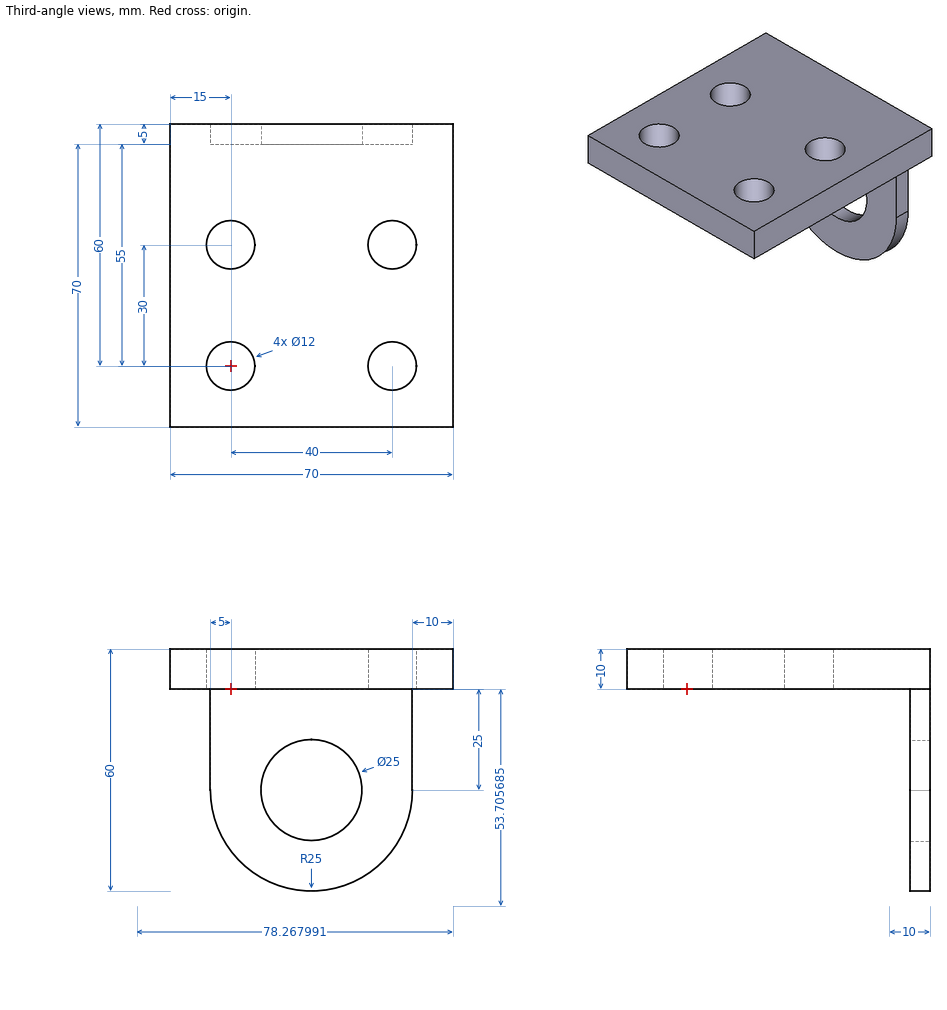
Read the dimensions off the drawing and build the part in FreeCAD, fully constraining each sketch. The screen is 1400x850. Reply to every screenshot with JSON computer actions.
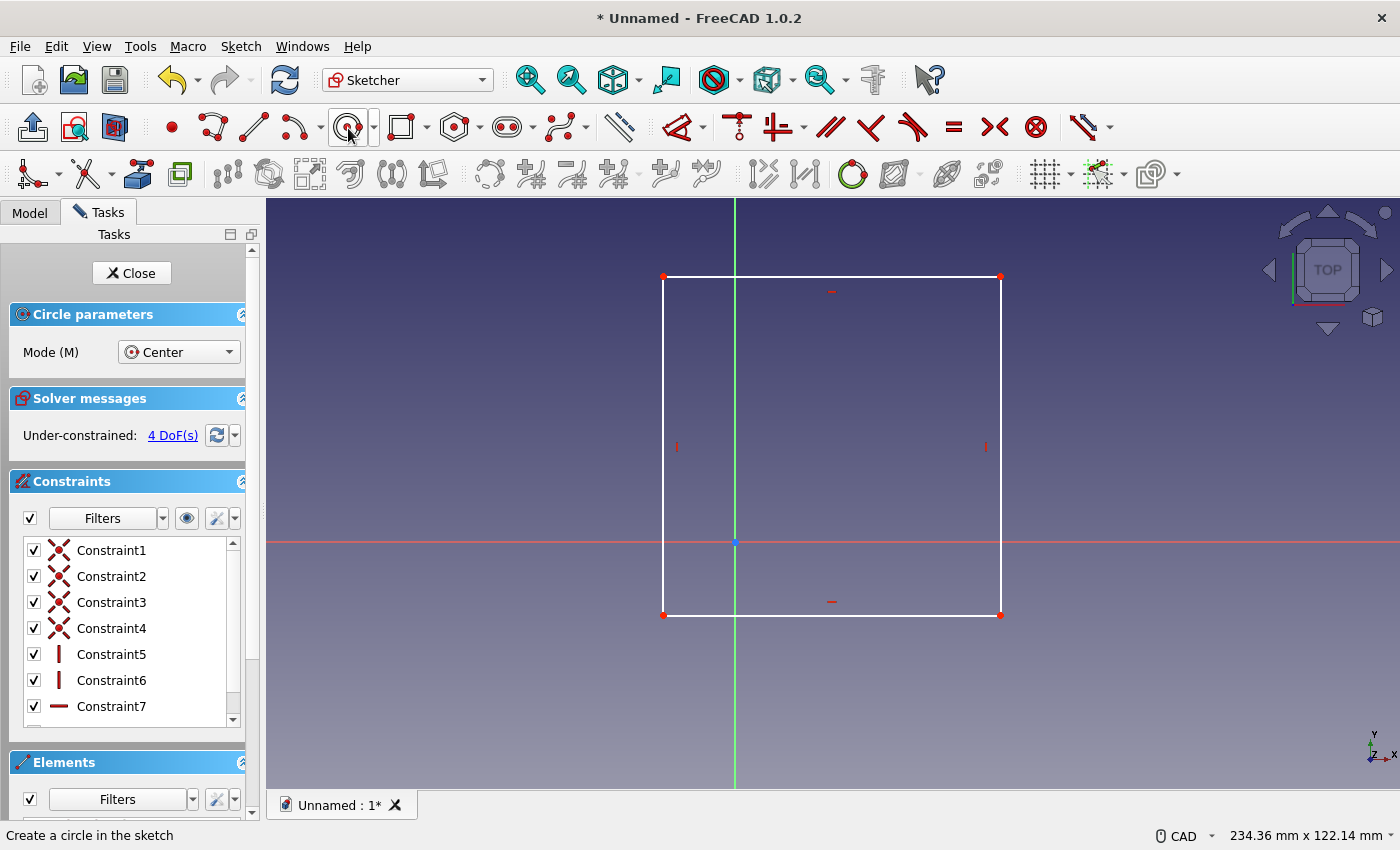
{"action": "left_click", "coordinate": [735, 542]}
{"action": "left_click", "coordinate": [756, 522]}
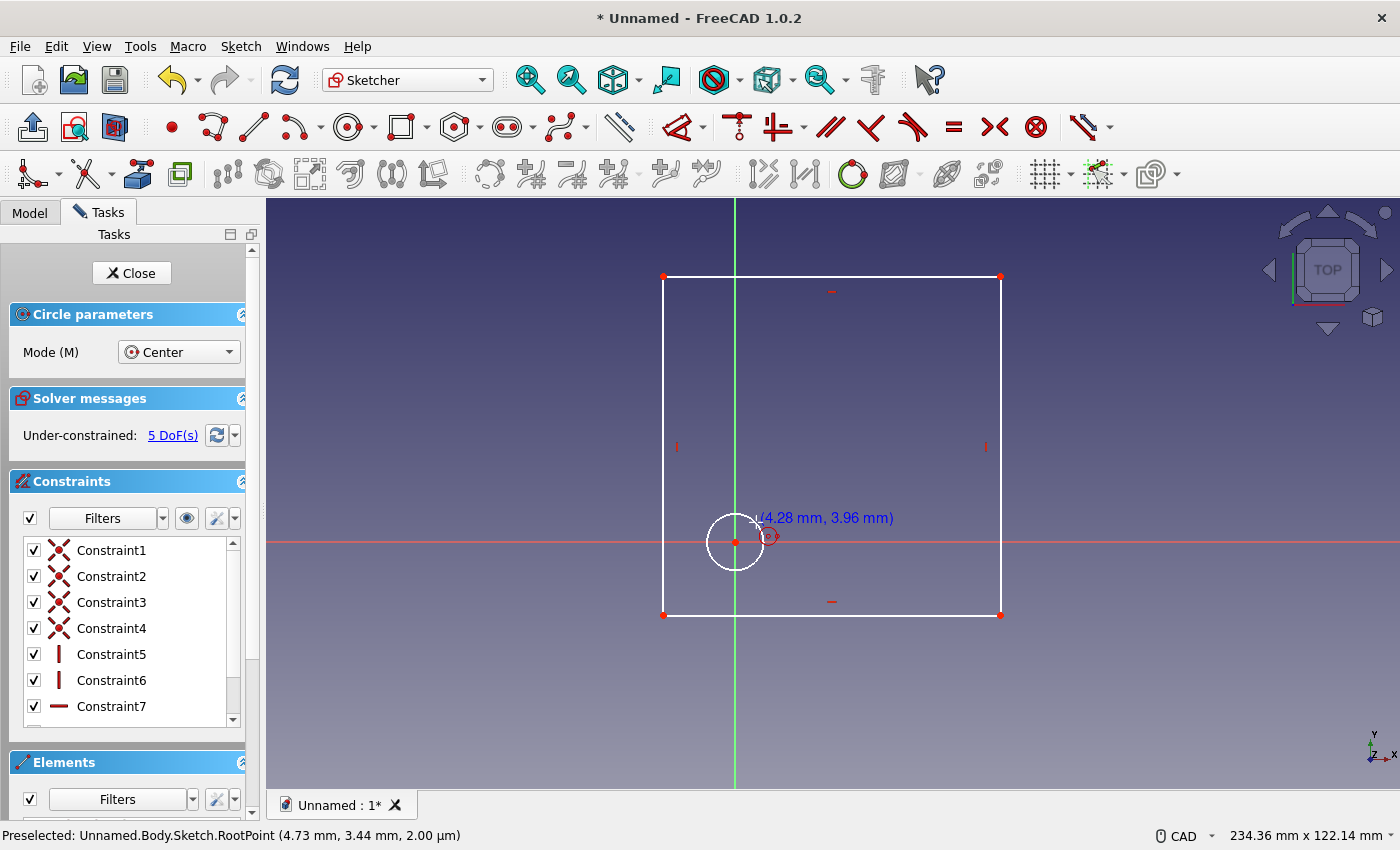
{"action": "left_click", "coordinate": [929, 542]}
{"action": "left_click", "coordinate": [949, 522]}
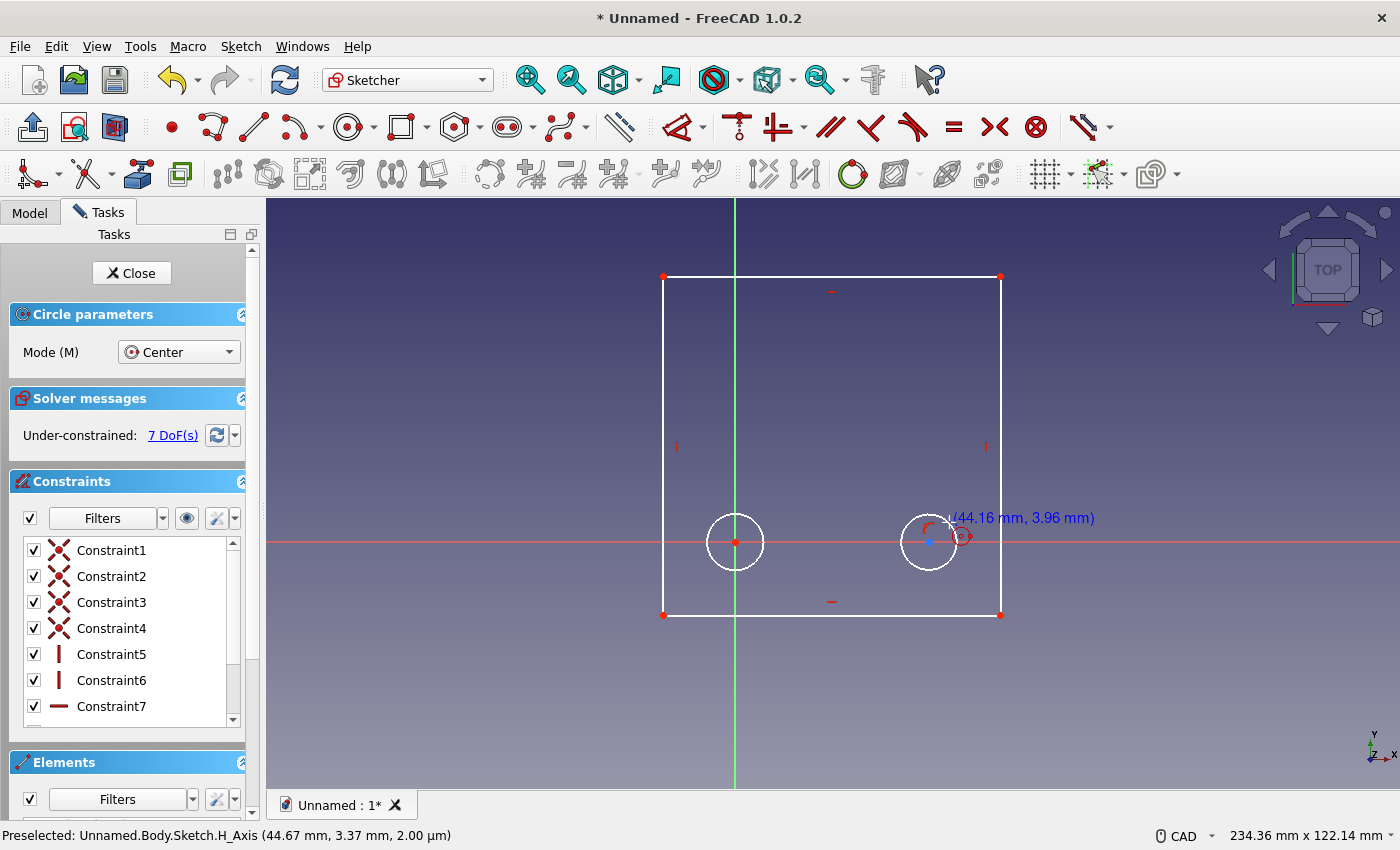
{"action": "left_click", "coordinate": [735, 397]}
{"action": "left_click", "coordinate": [756, 376]}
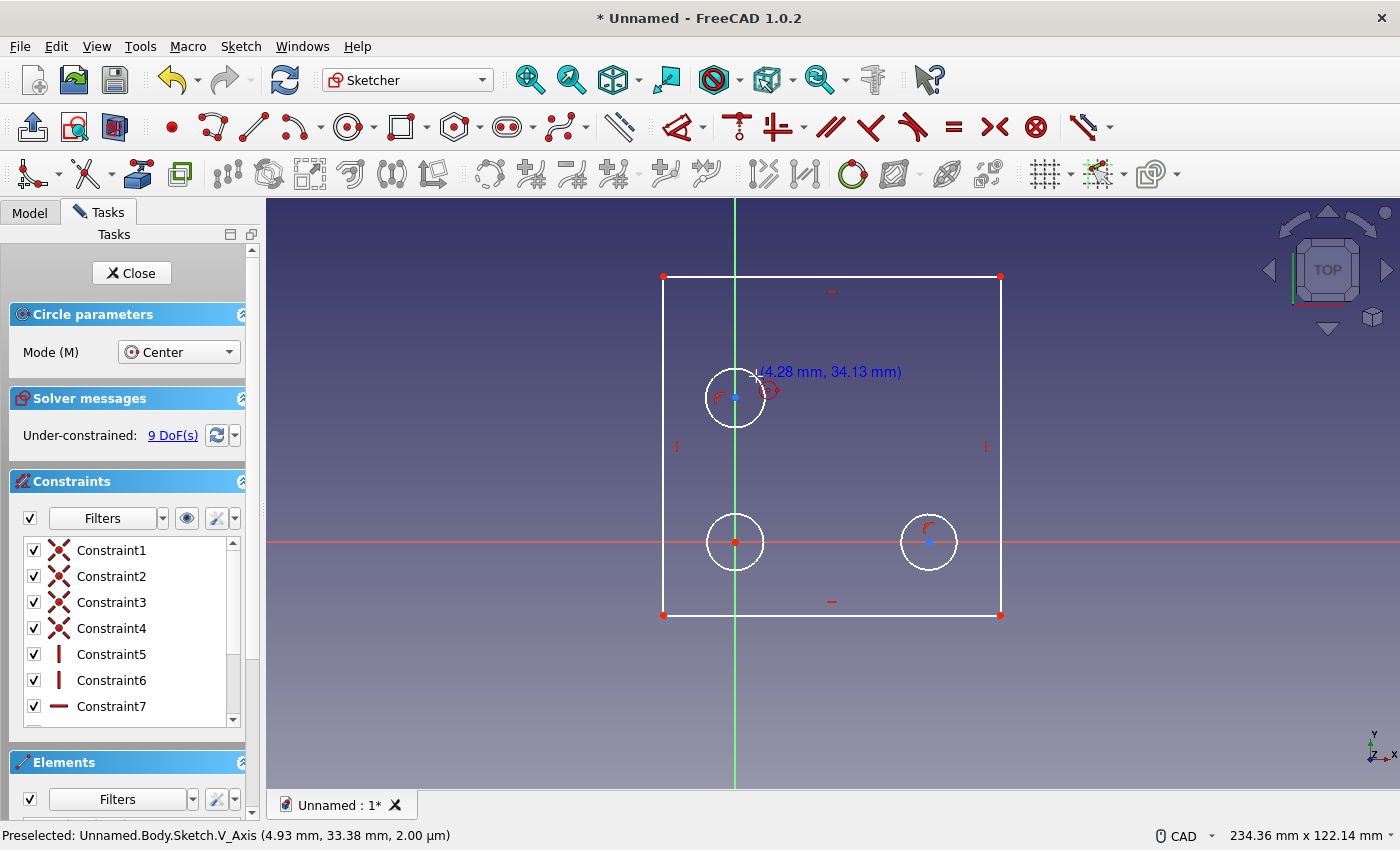
{"action": "left_click", "coordinate": [929, 397]}
{"action": "left_click", "coordinate": [949, 376]}
{"action": "key", "text": "Escape"}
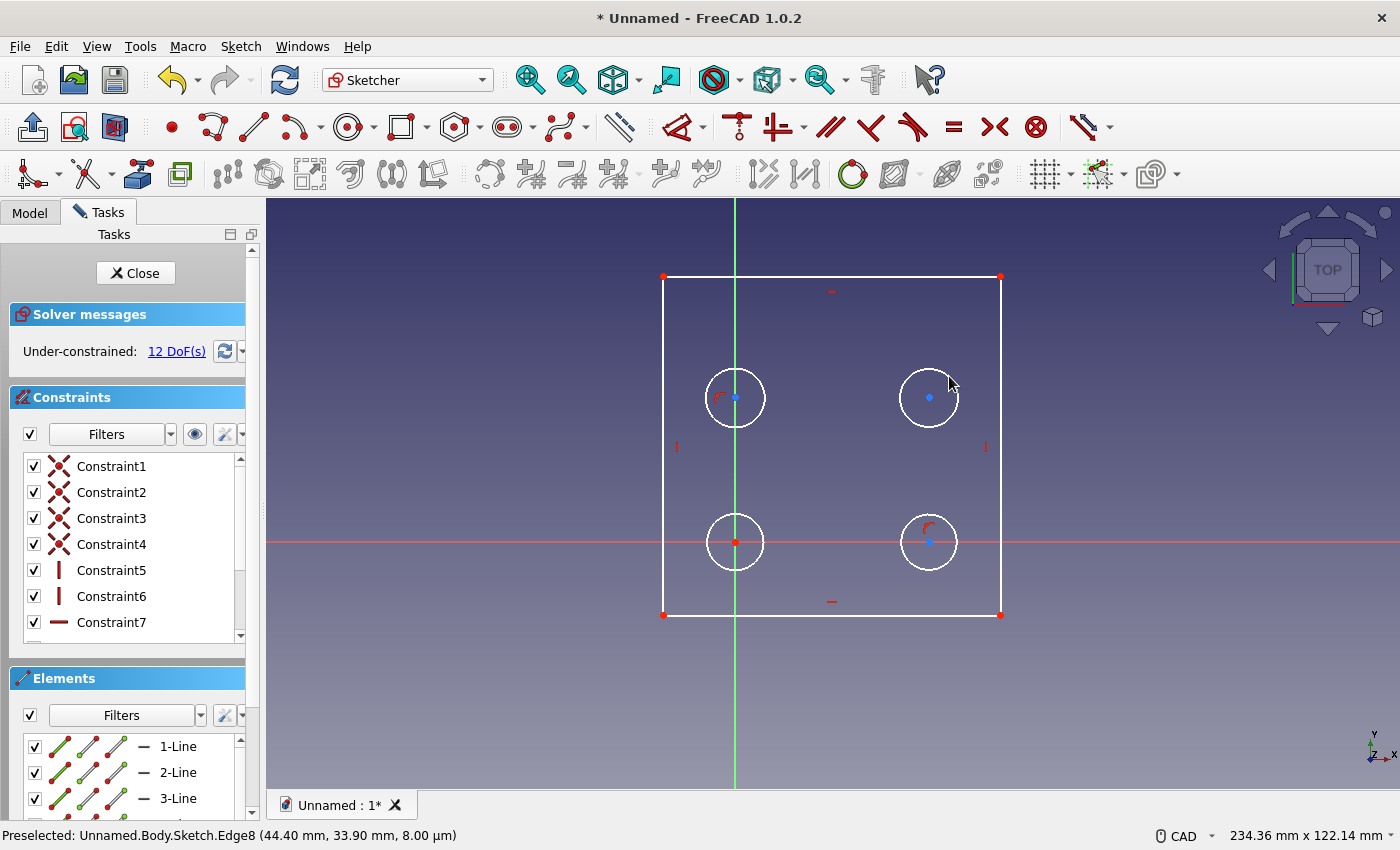
{"action": "left_click", "coordinate": [755, 522]}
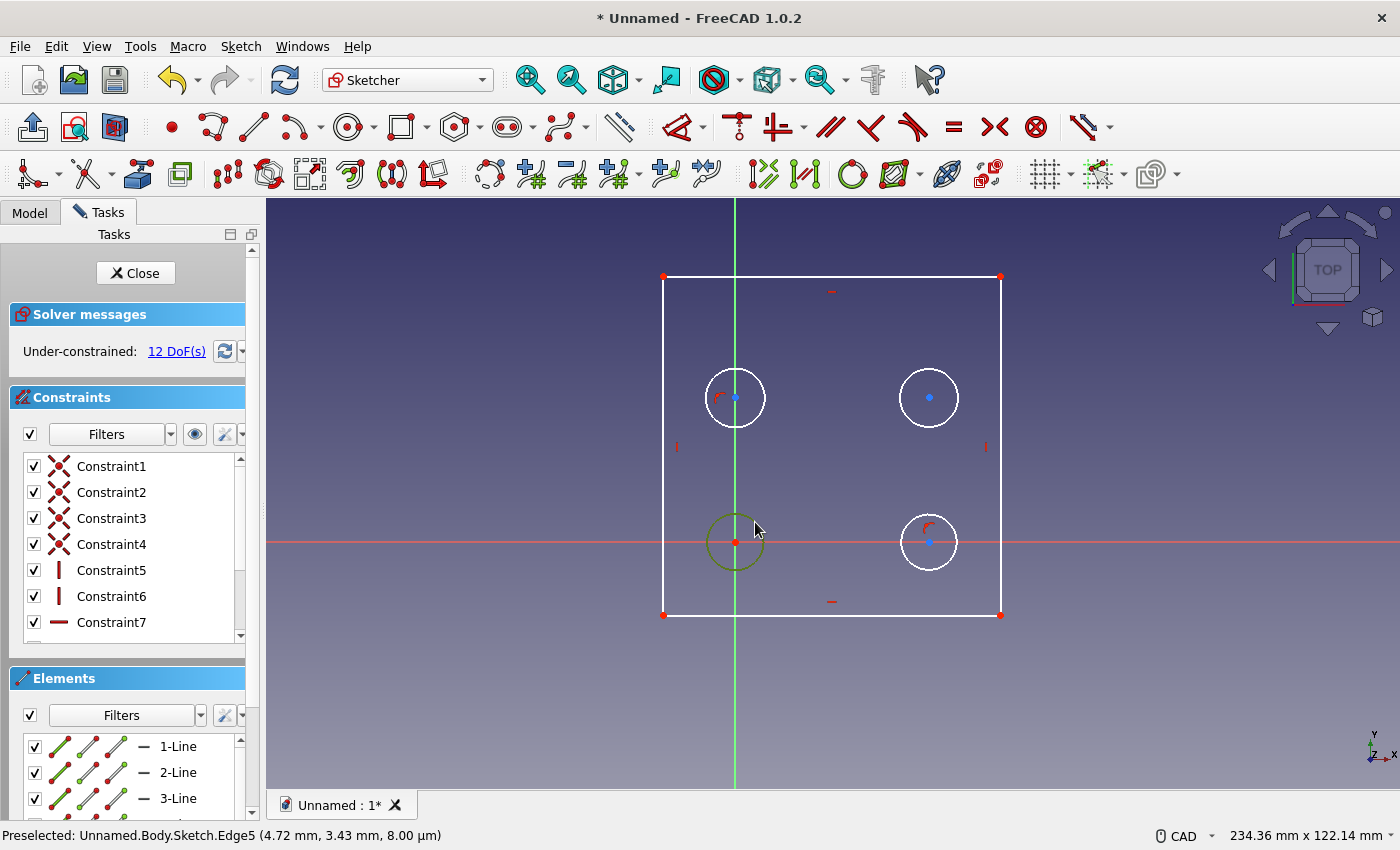
{"action": "left_click", "coordinate": [949, 523]}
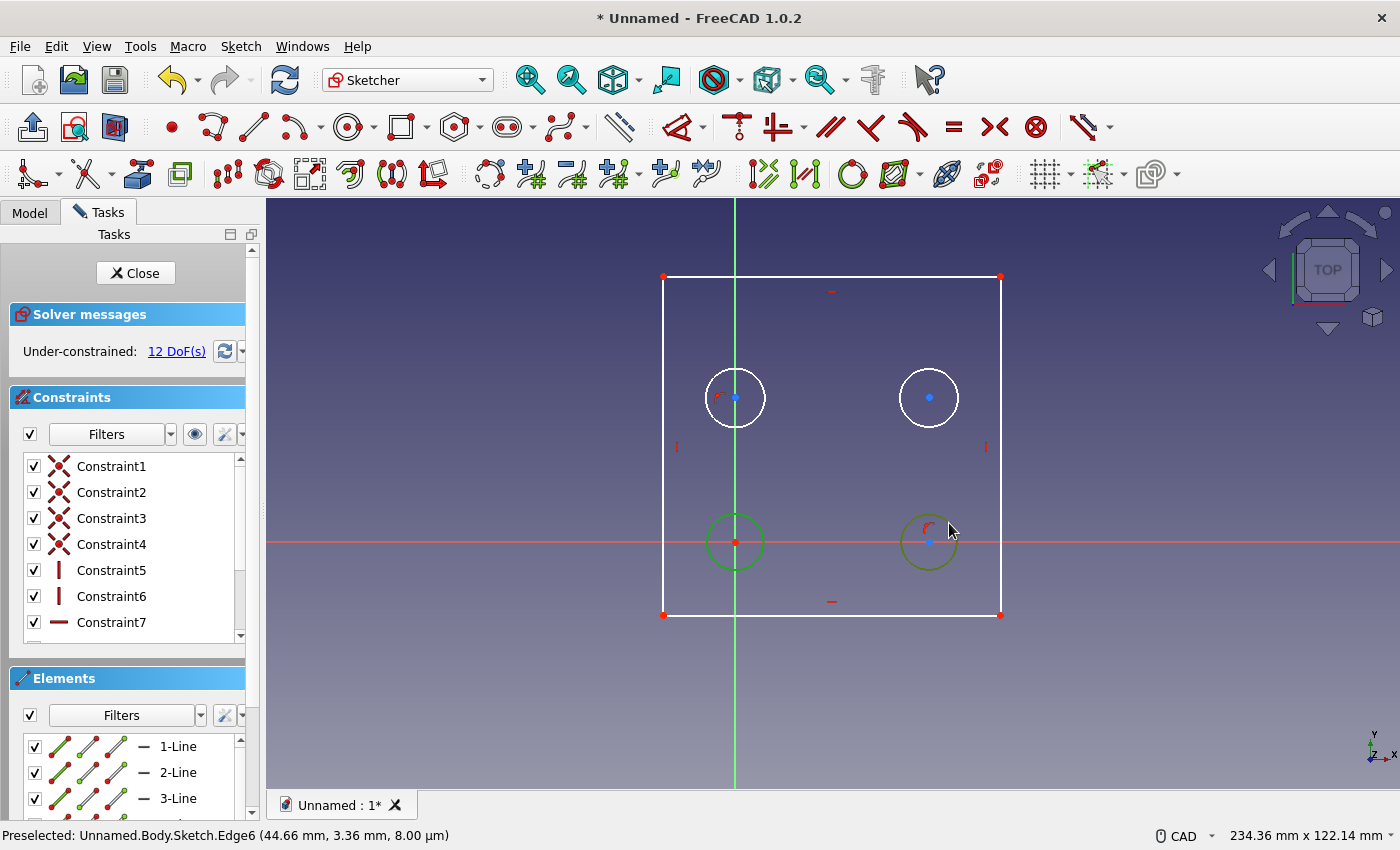
{"action": "left_click", "coordinate": [756, 377]}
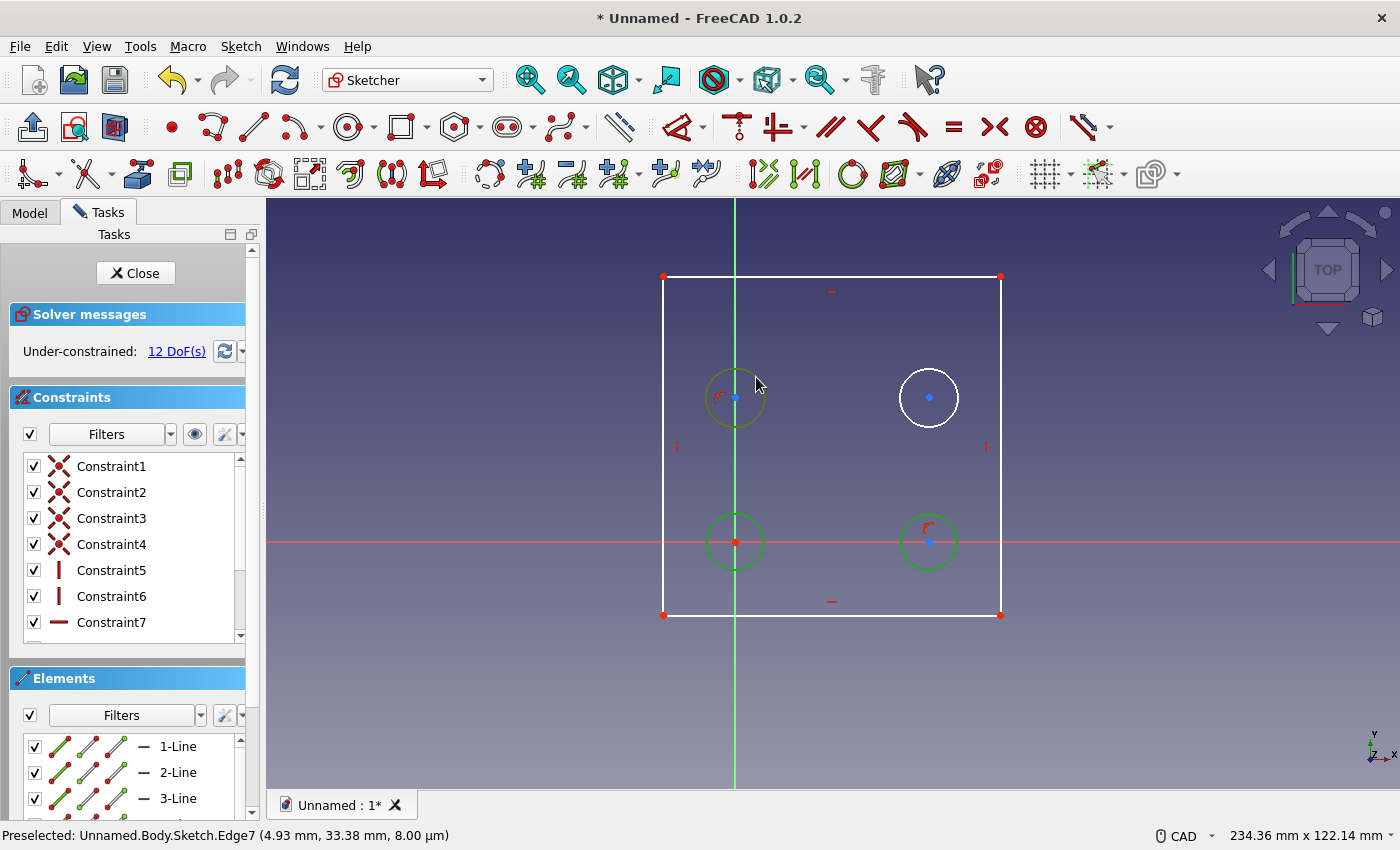
{"action": "left_click", "coordinate": [949, 377]}